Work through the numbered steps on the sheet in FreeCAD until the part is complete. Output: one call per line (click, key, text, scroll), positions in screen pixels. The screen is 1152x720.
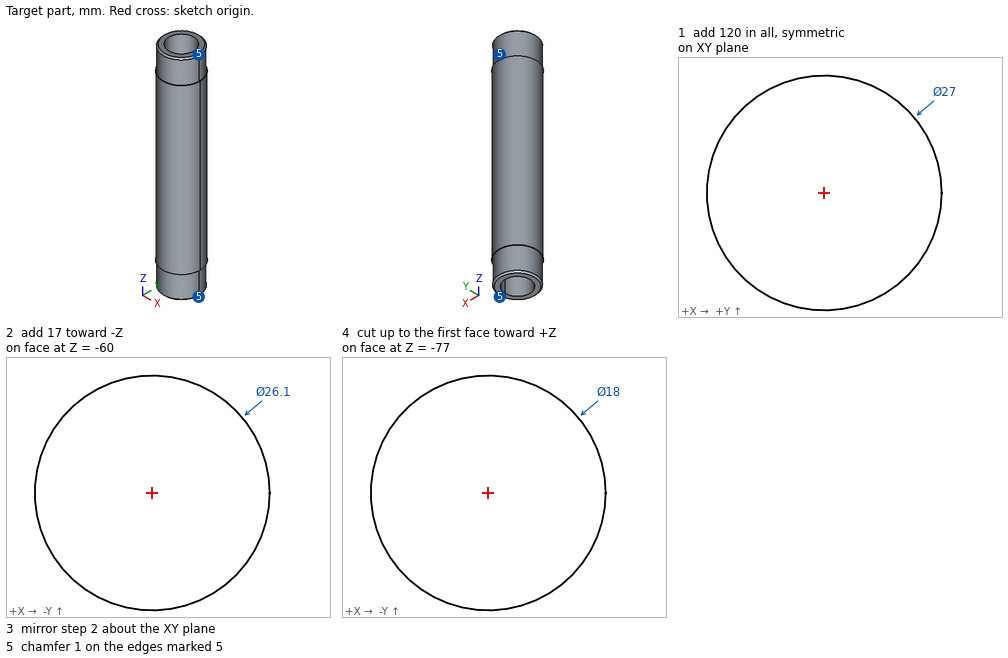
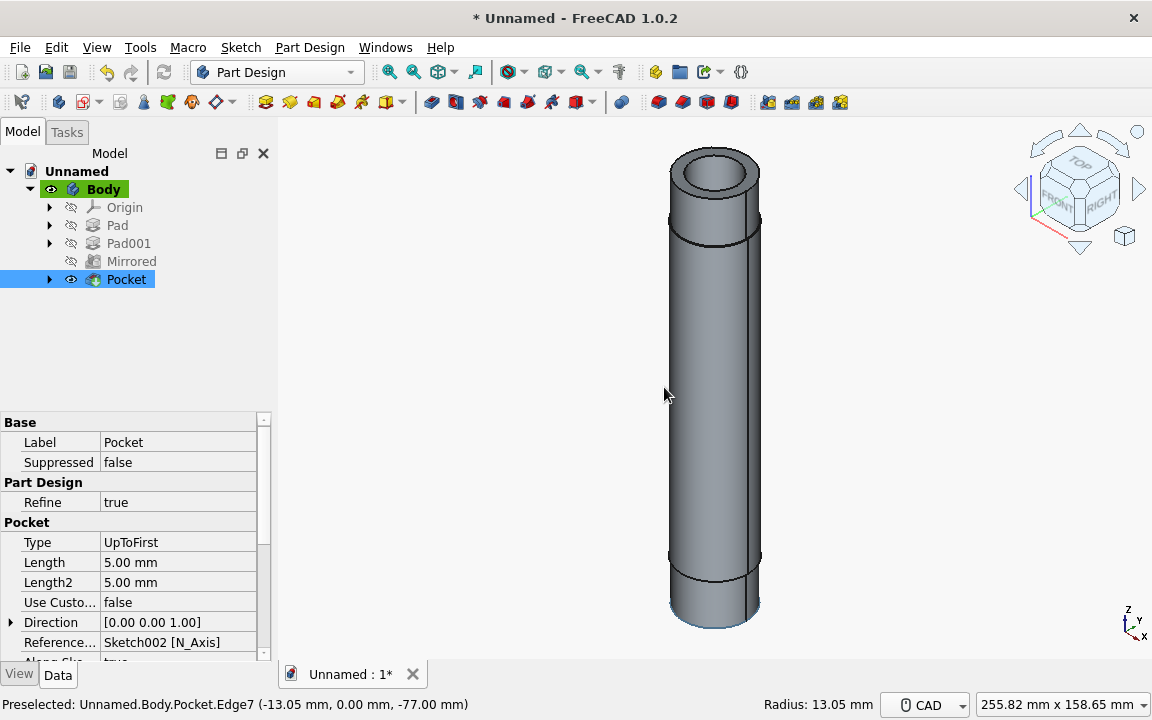
click(683, 154, ctrl)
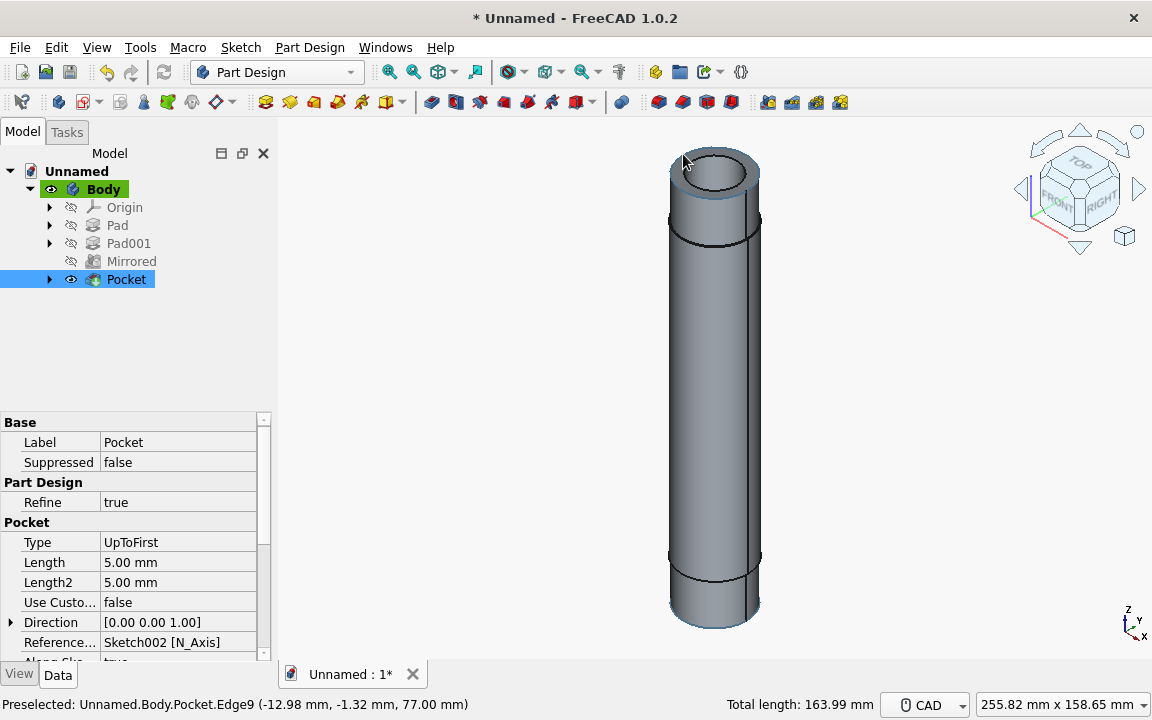
click(684, 102)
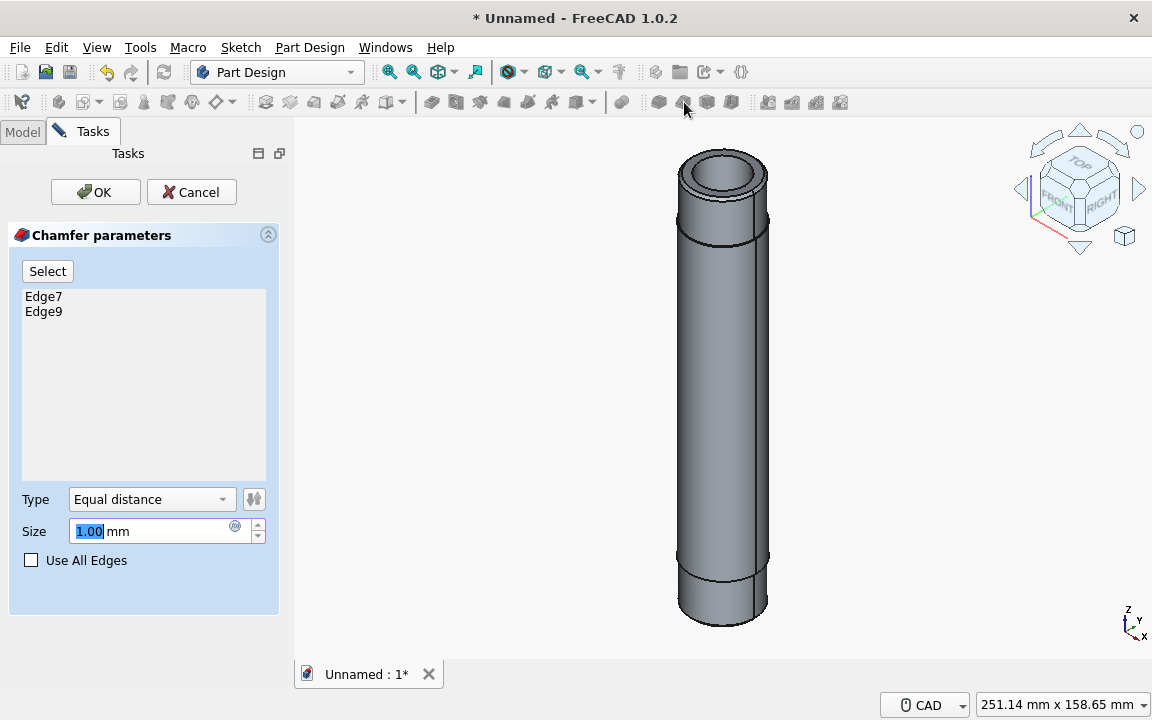
text(1)
key(Tab)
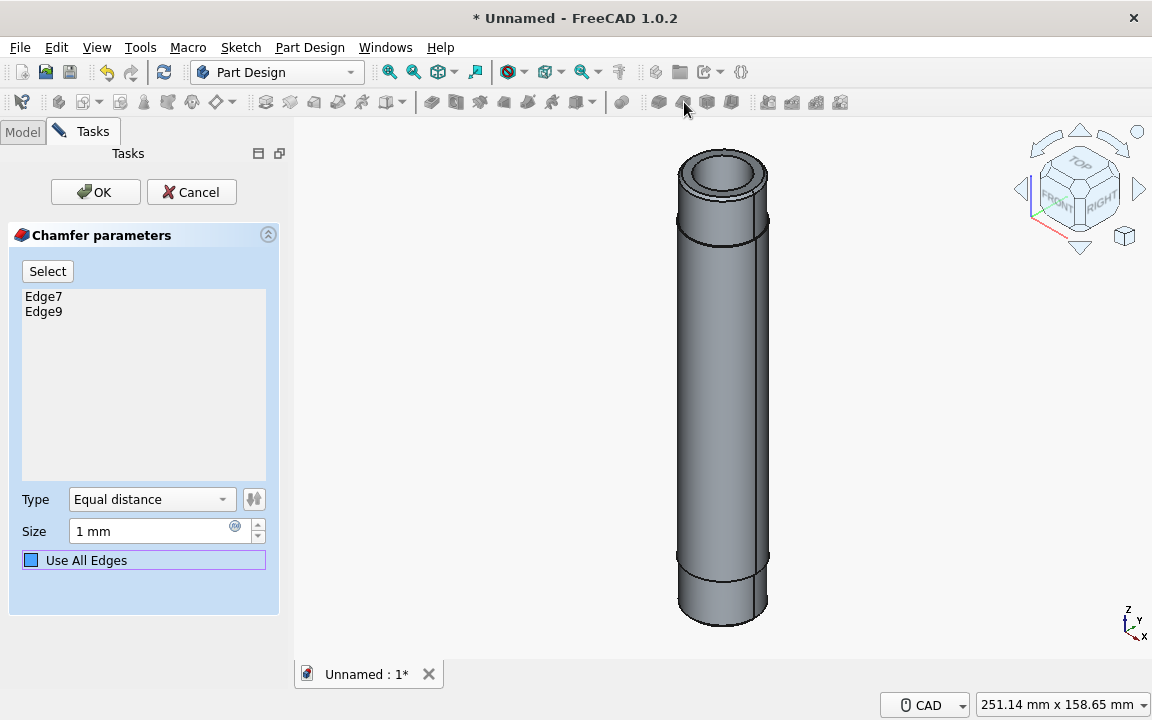
click(96, 192)